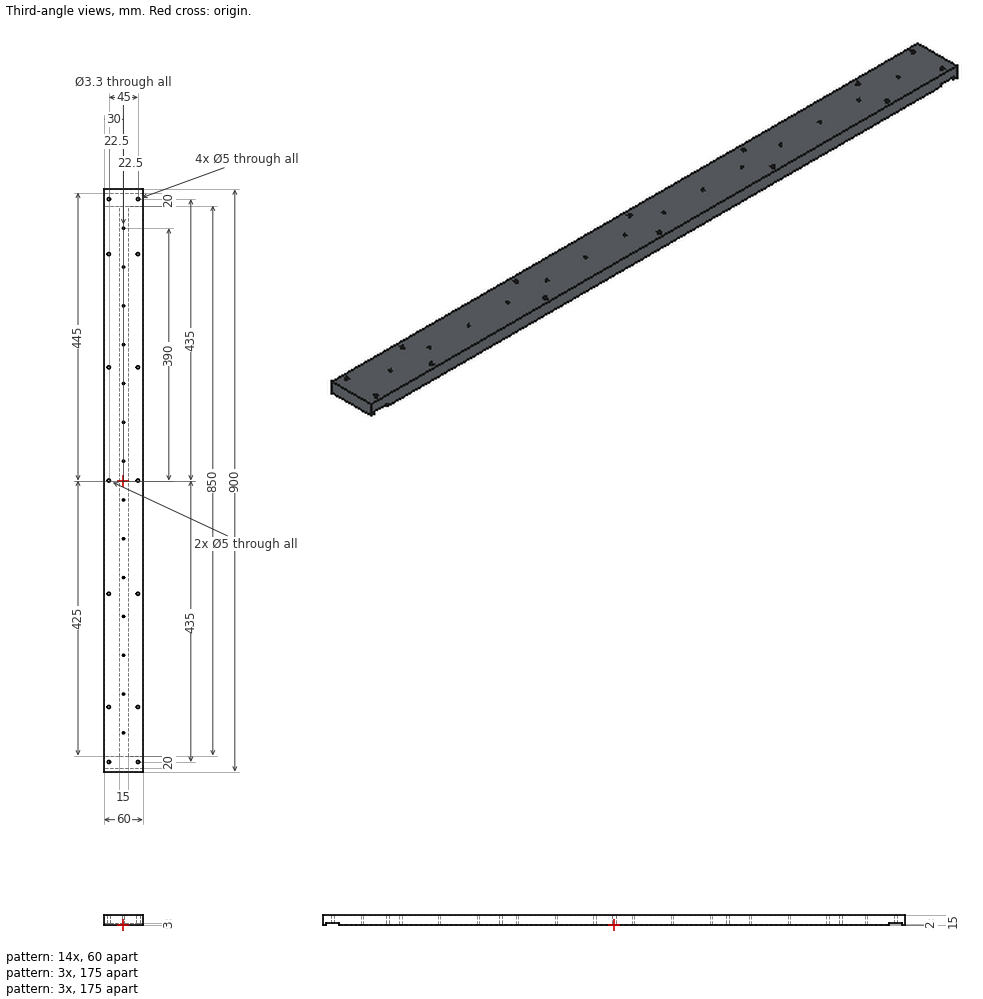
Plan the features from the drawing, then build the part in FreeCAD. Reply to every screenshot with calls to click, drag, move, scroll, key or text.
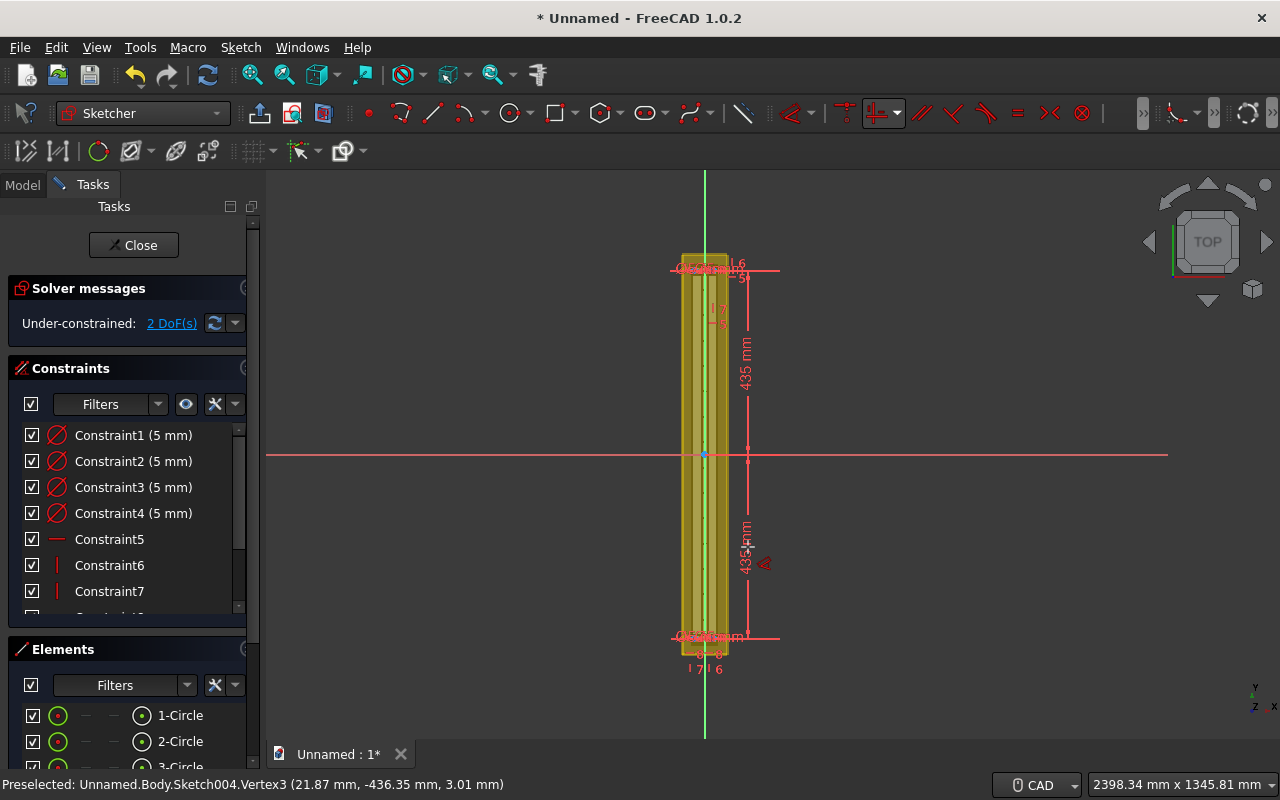
scroll(714, 271, up, 4)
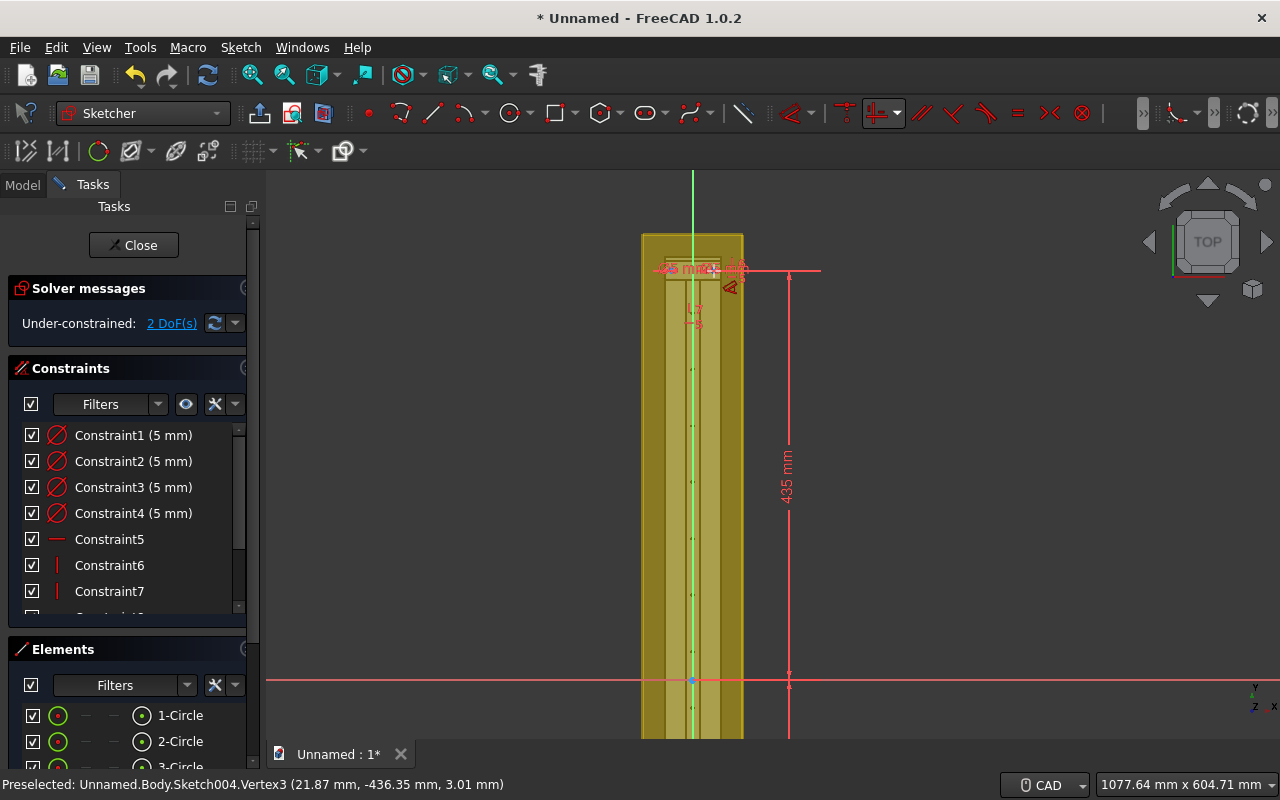
click(713, 271)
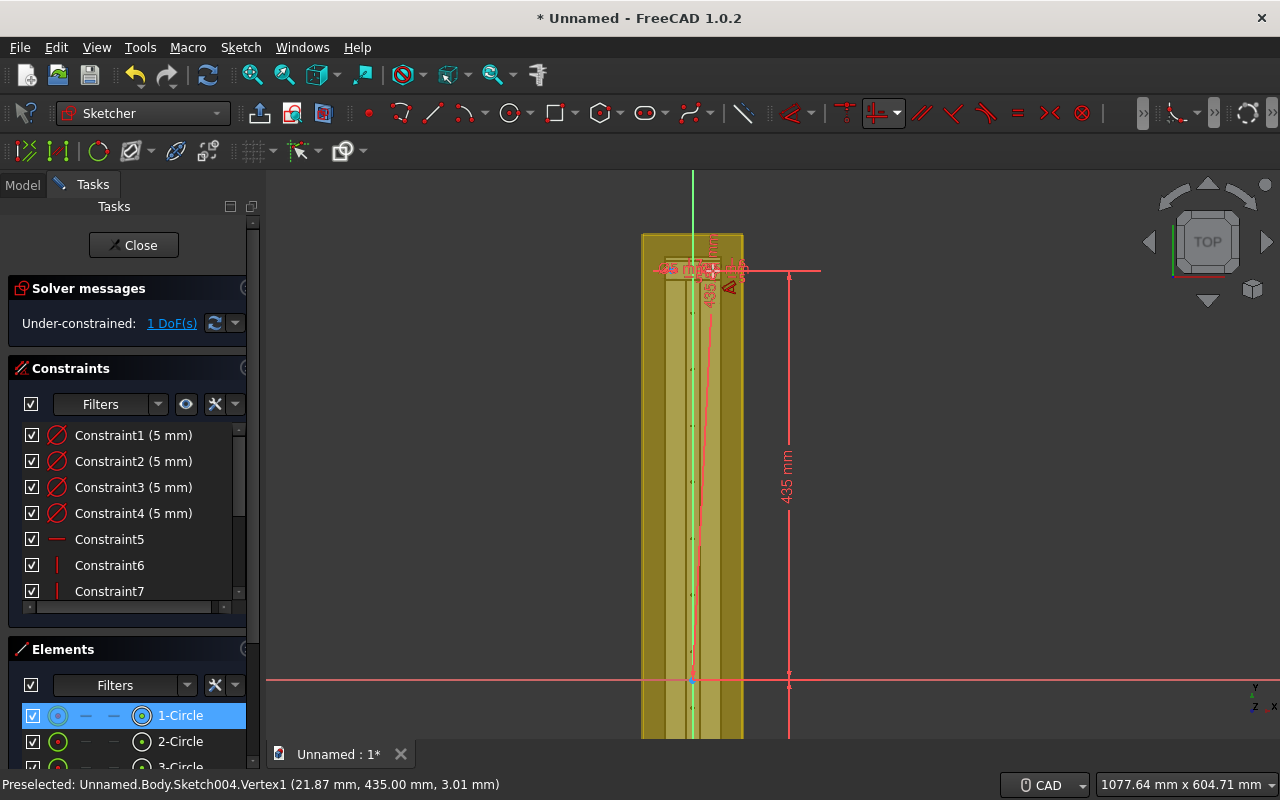
click(671, 271)
click(677, 237)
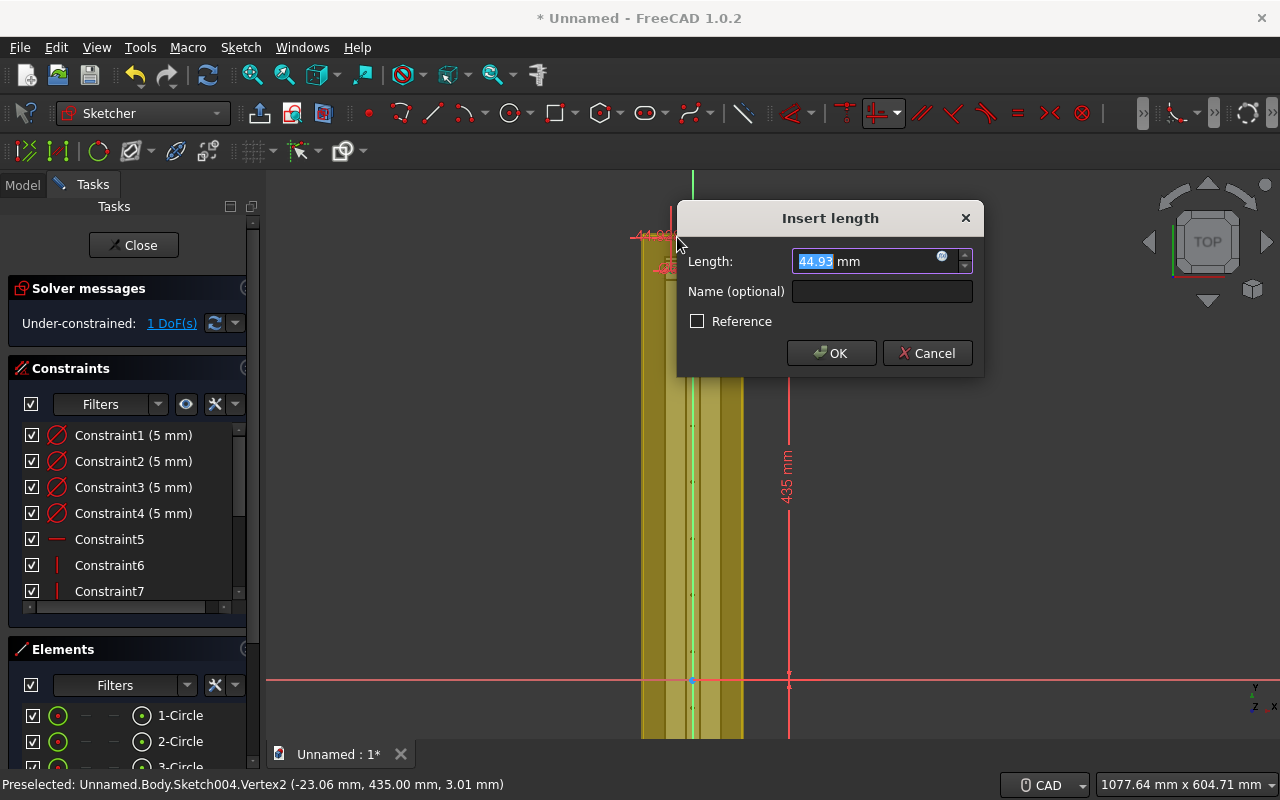
text(45)
key(Return)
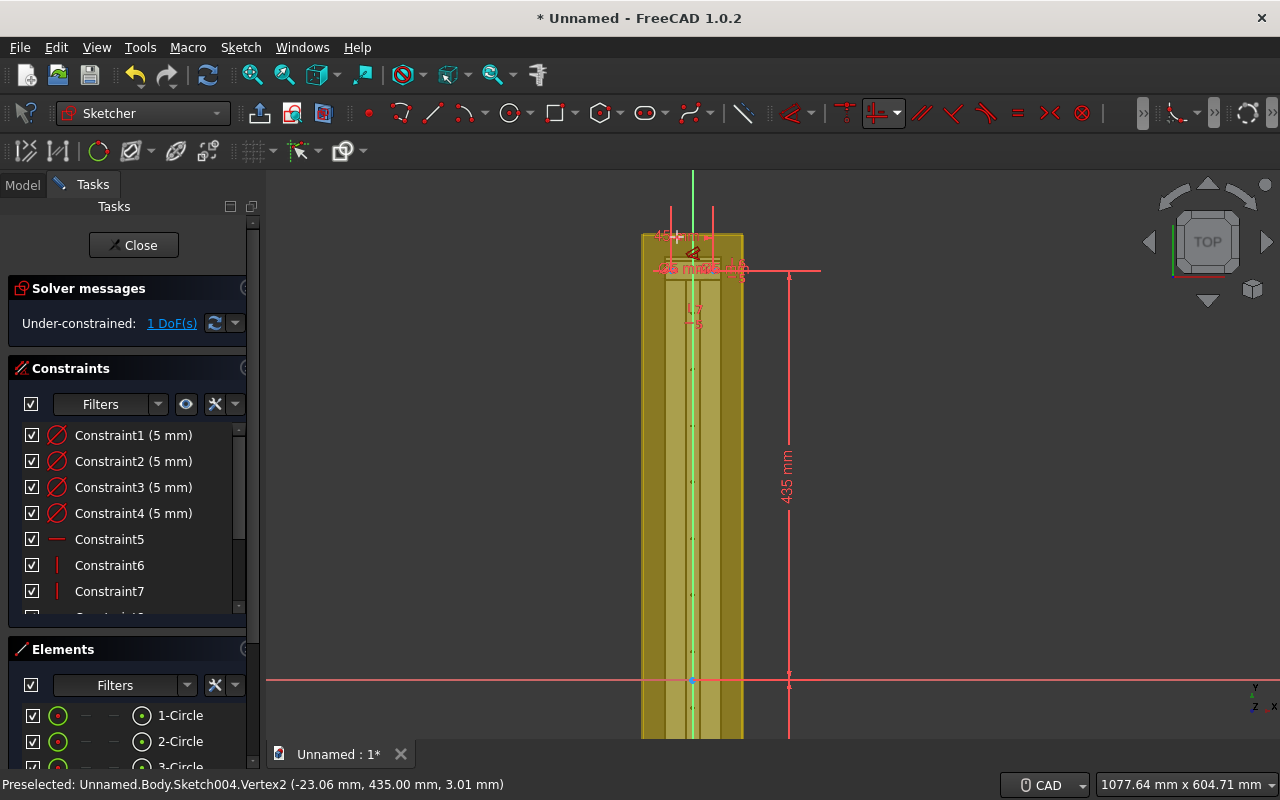
scroll(713, 271, up, 4)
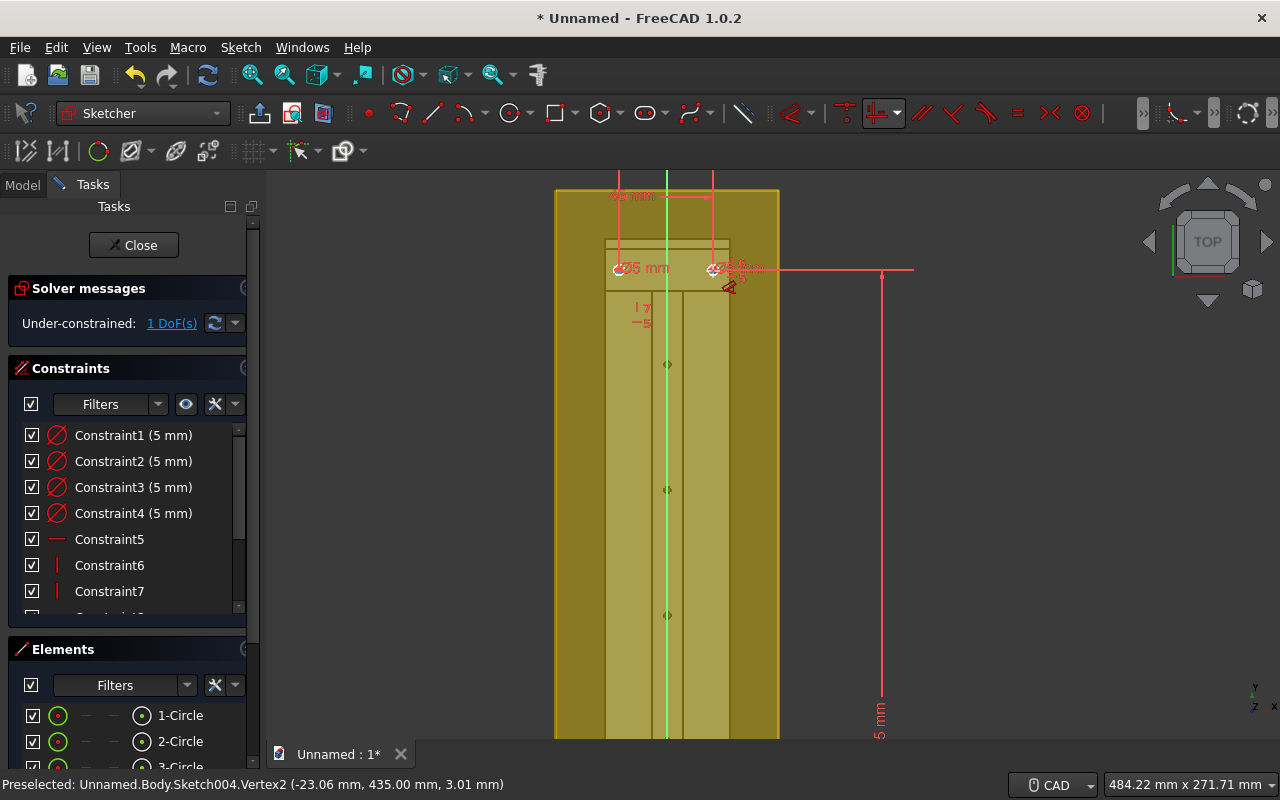
click(713, 270)
click(690, 236)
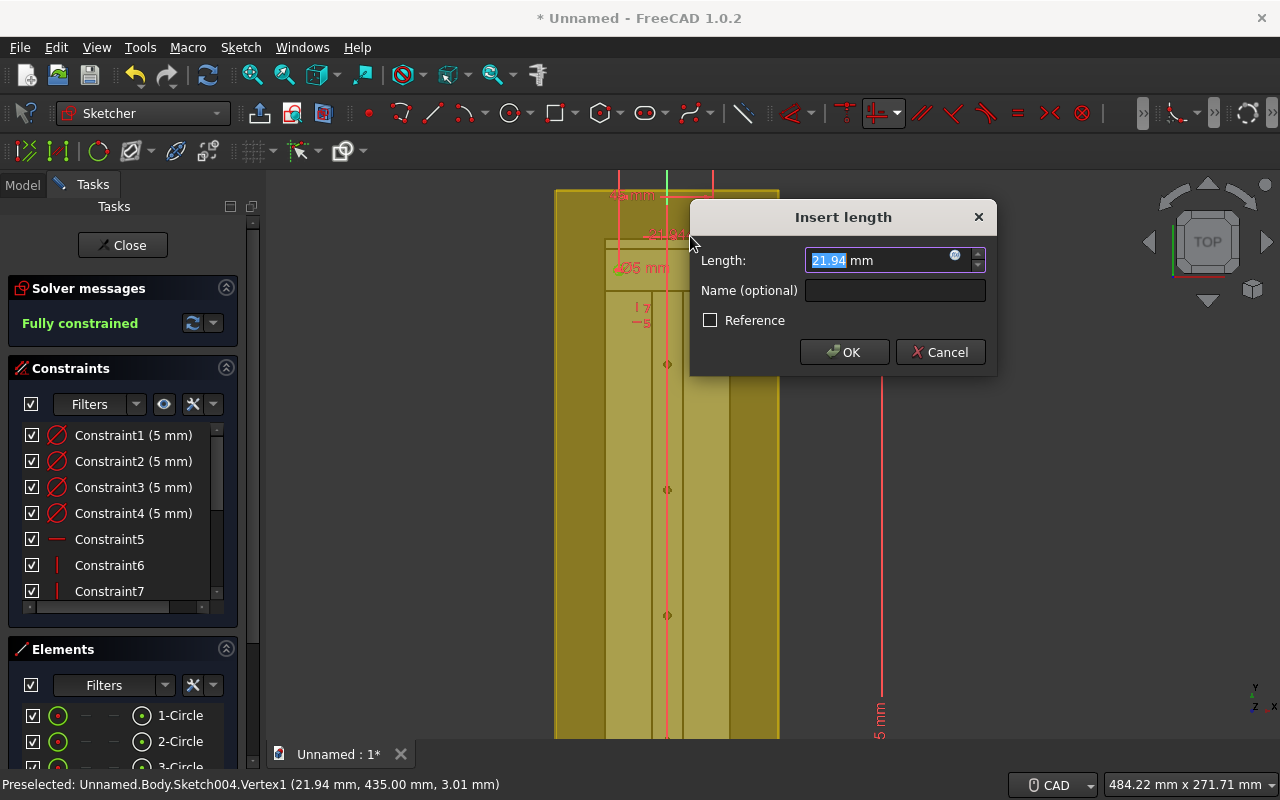
text(22.5)
key(Return)
key(Escape)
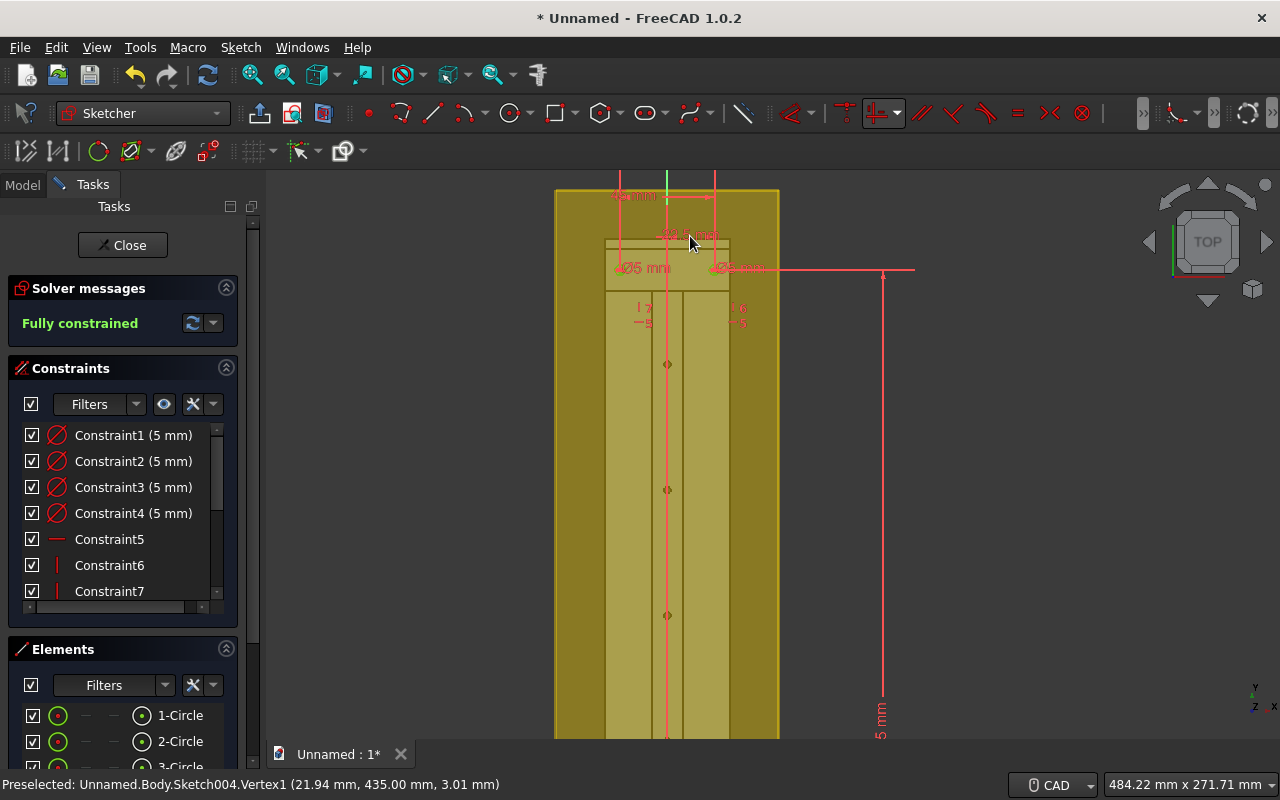
click(123, 245)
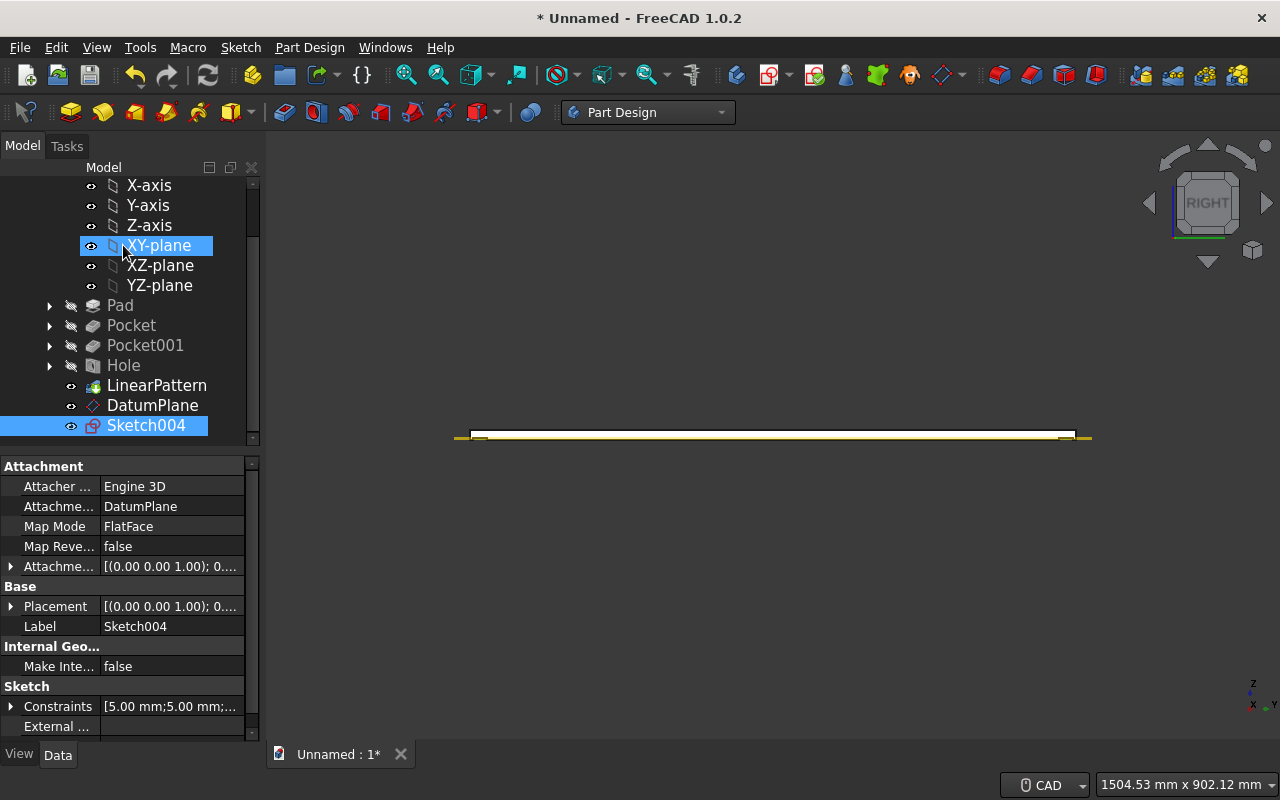
click(318, 112)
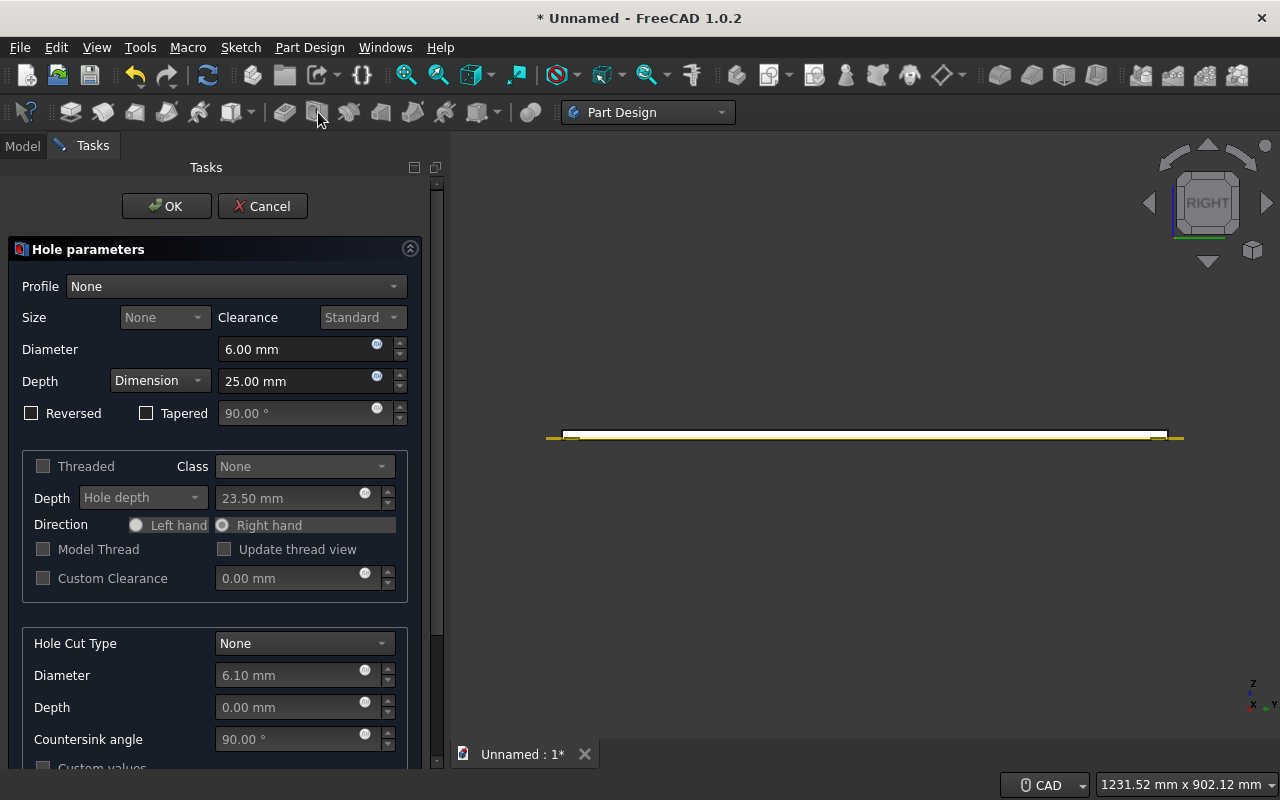
triple_click(305, 349)